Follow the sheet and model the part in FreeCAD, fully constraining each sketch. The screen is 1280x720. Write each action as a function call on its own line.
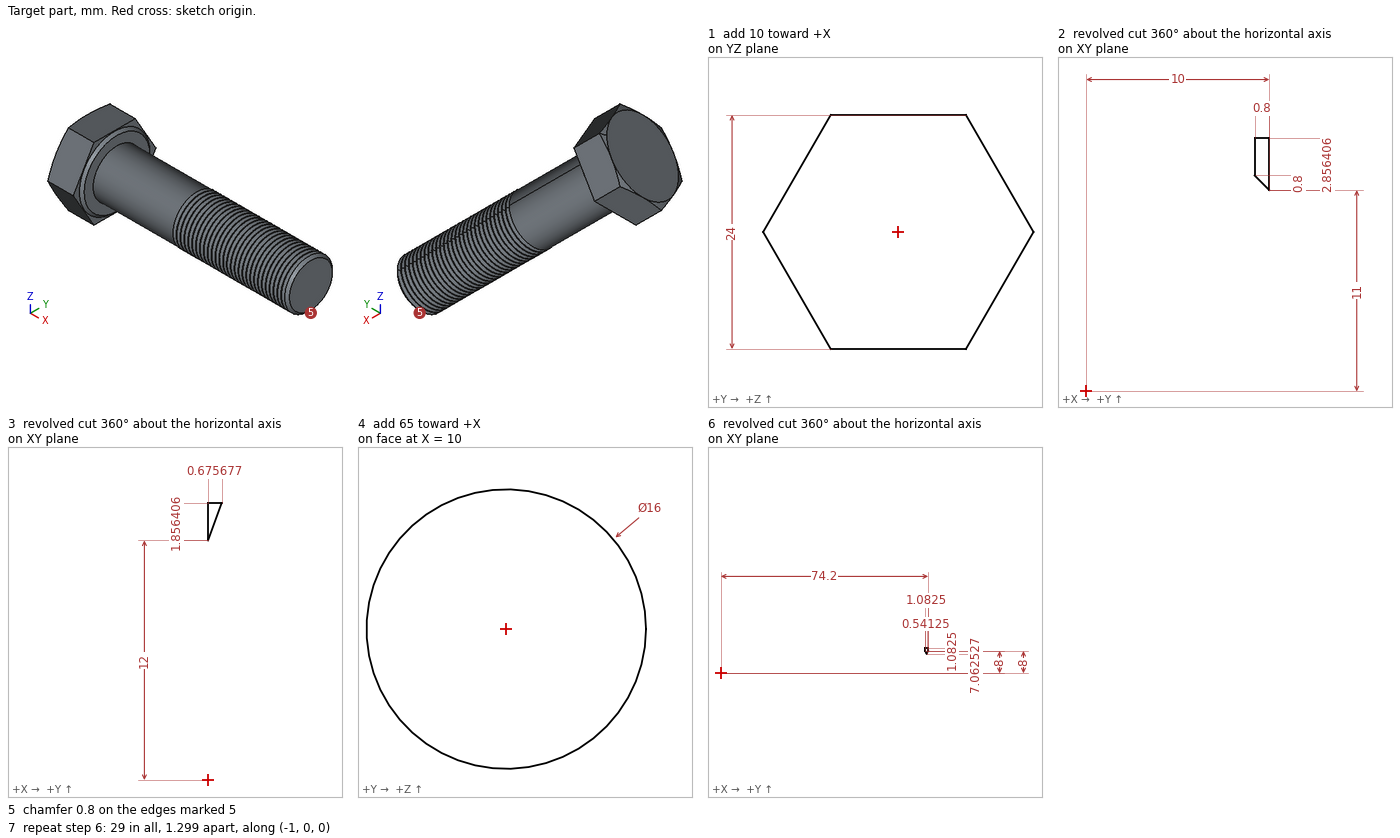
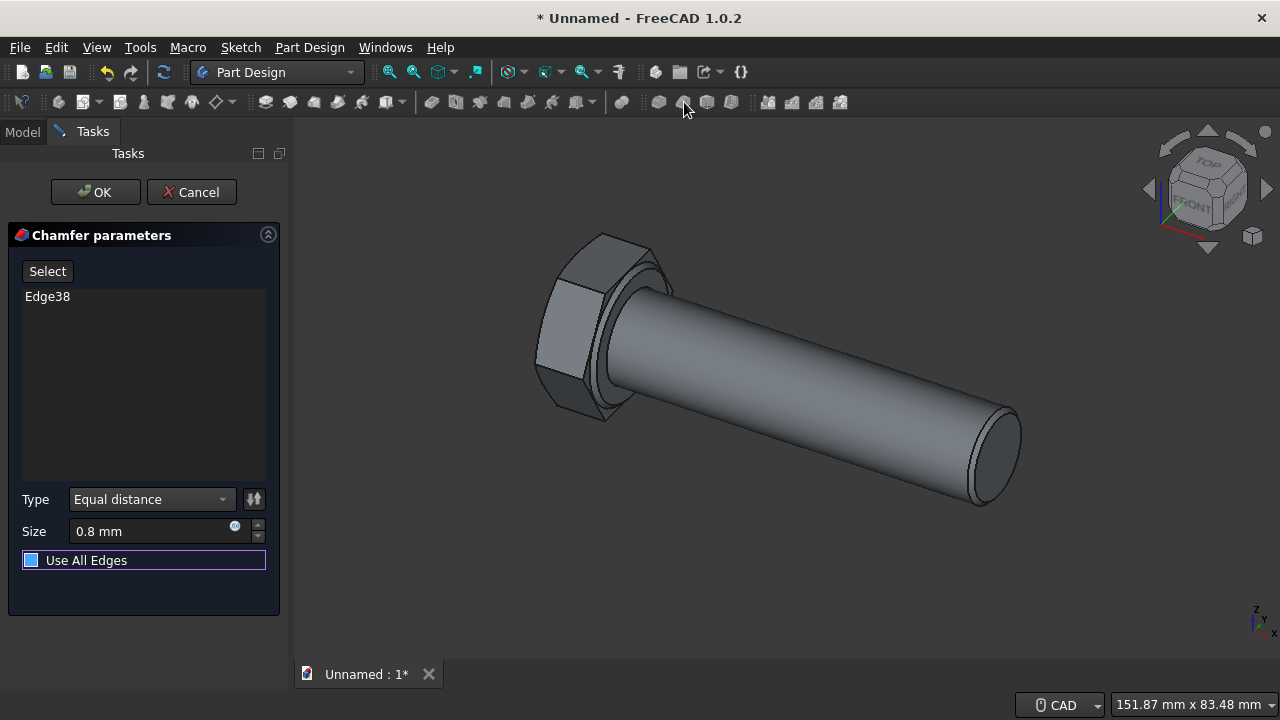
click(96, 192)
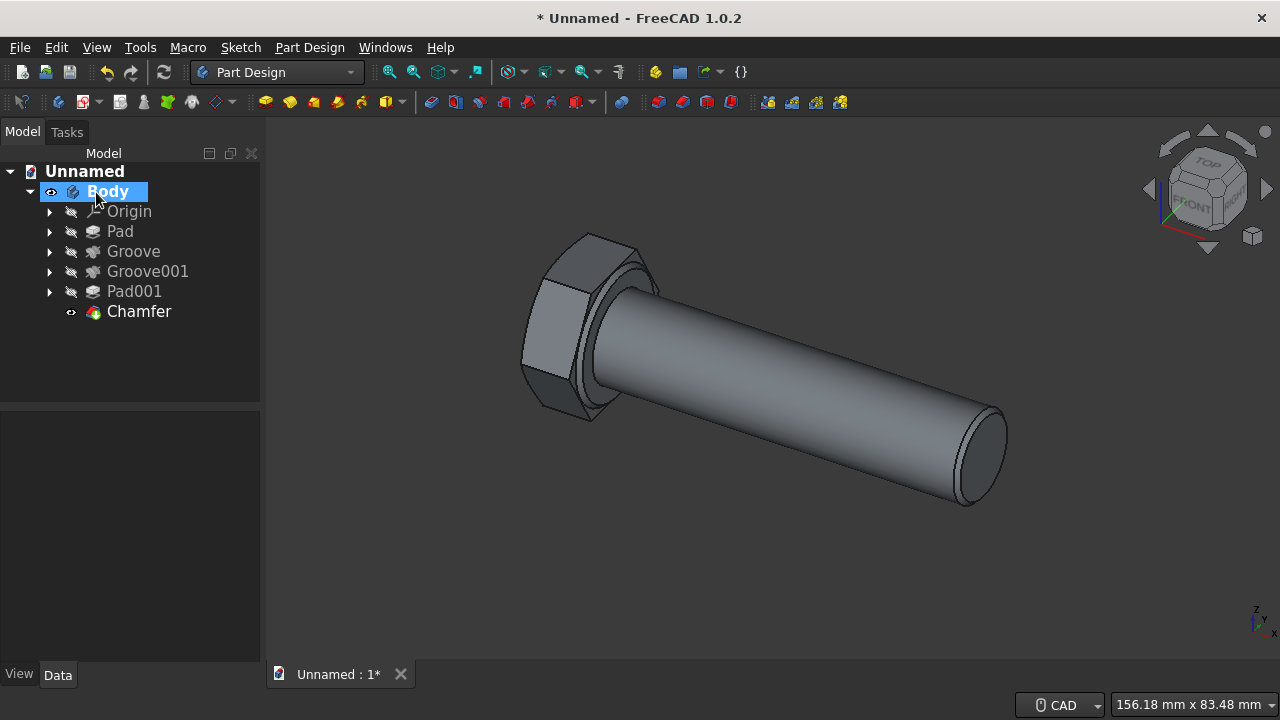
click(84, 102)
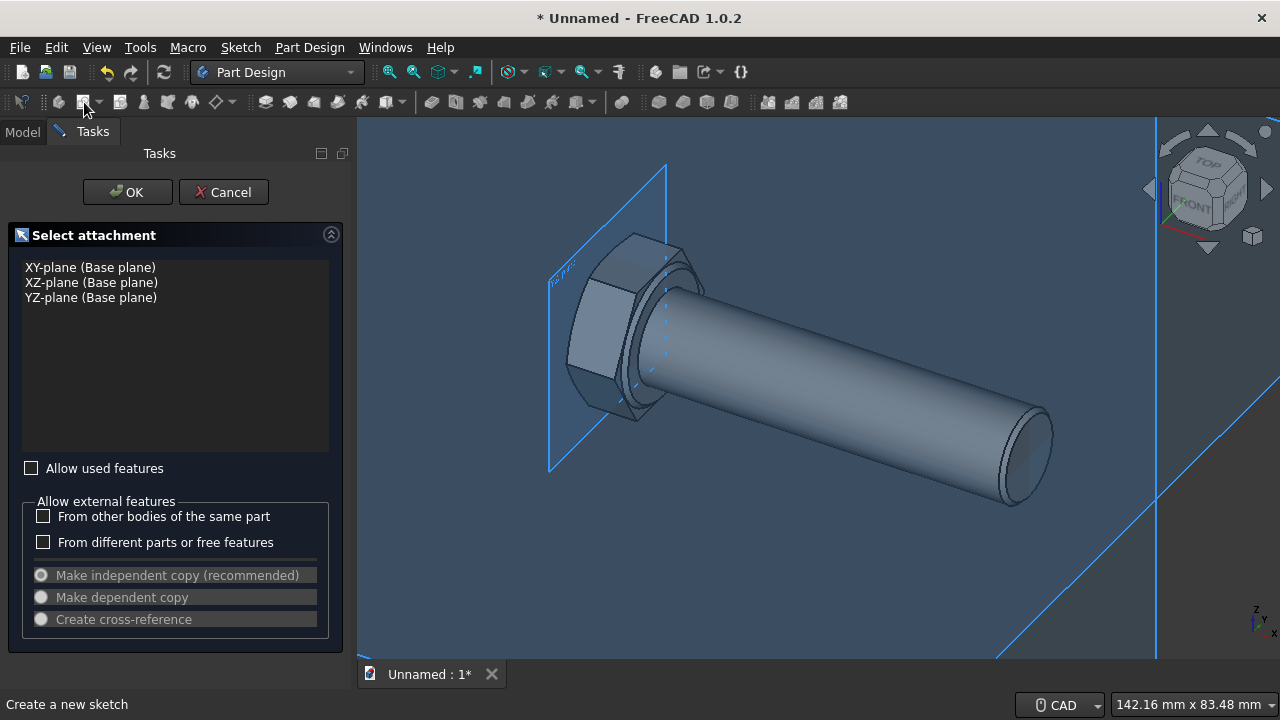
click(82, 268)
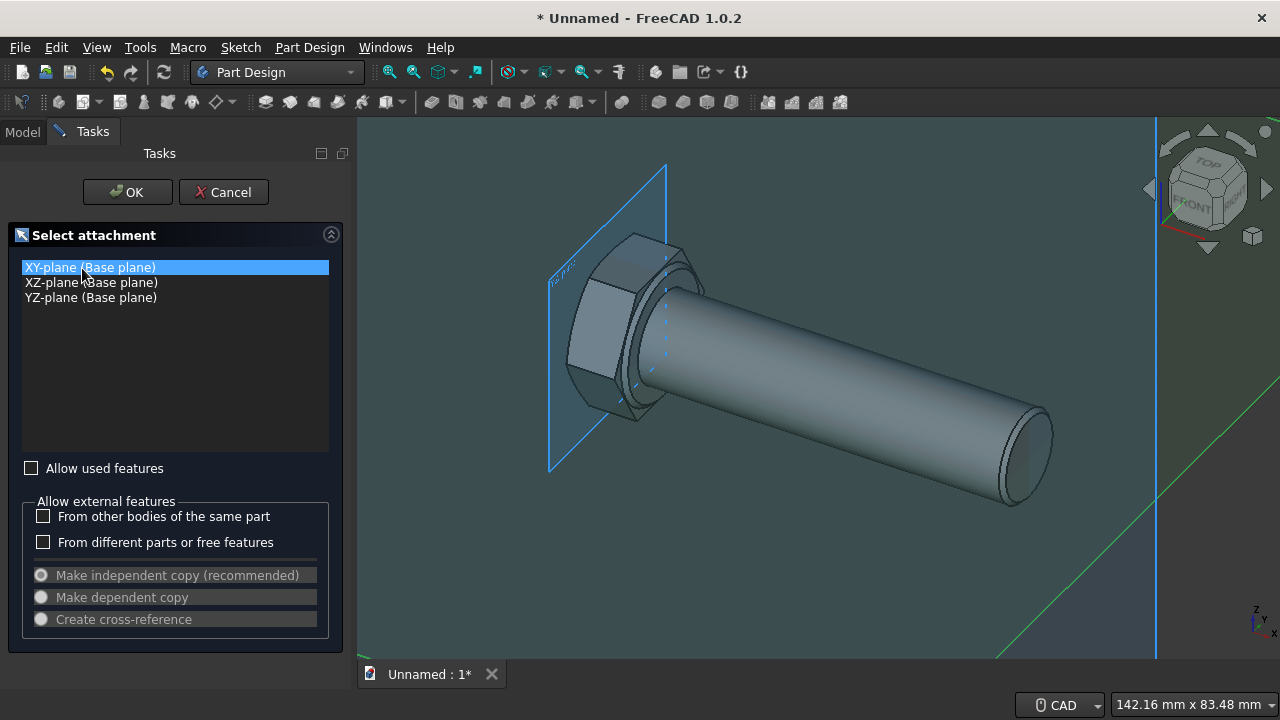
click(128, 192)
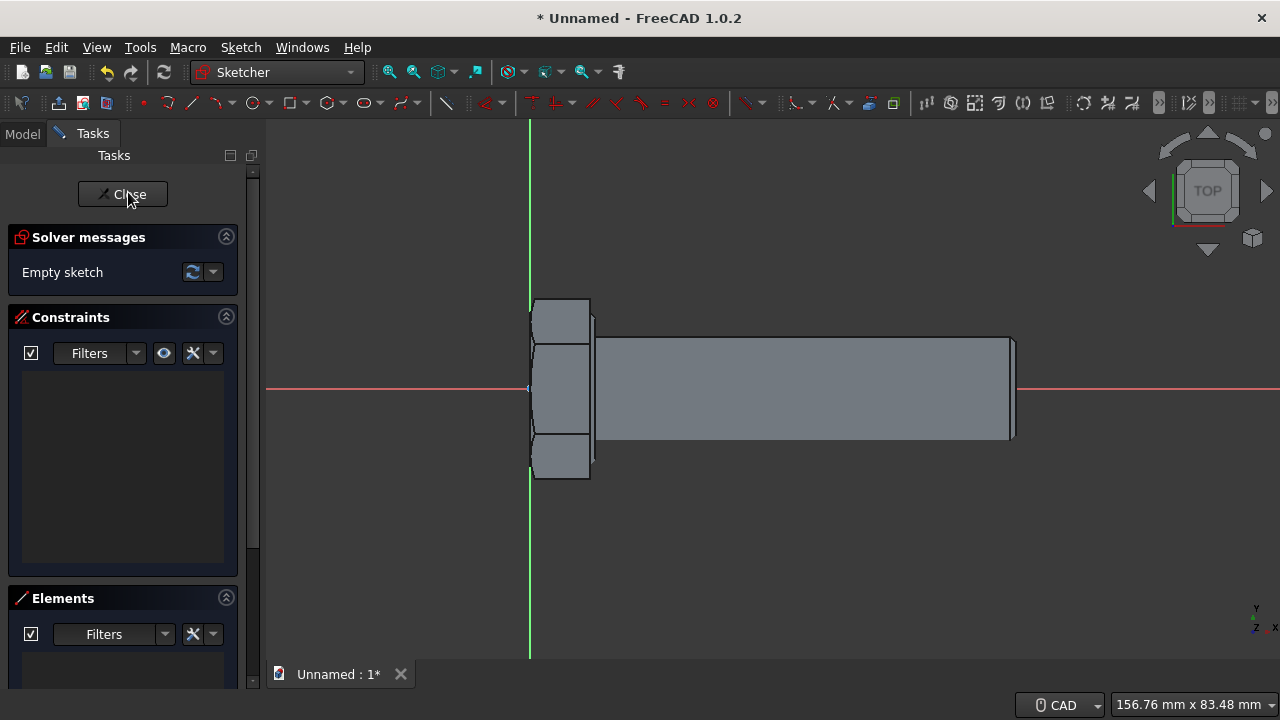
click(108, 104)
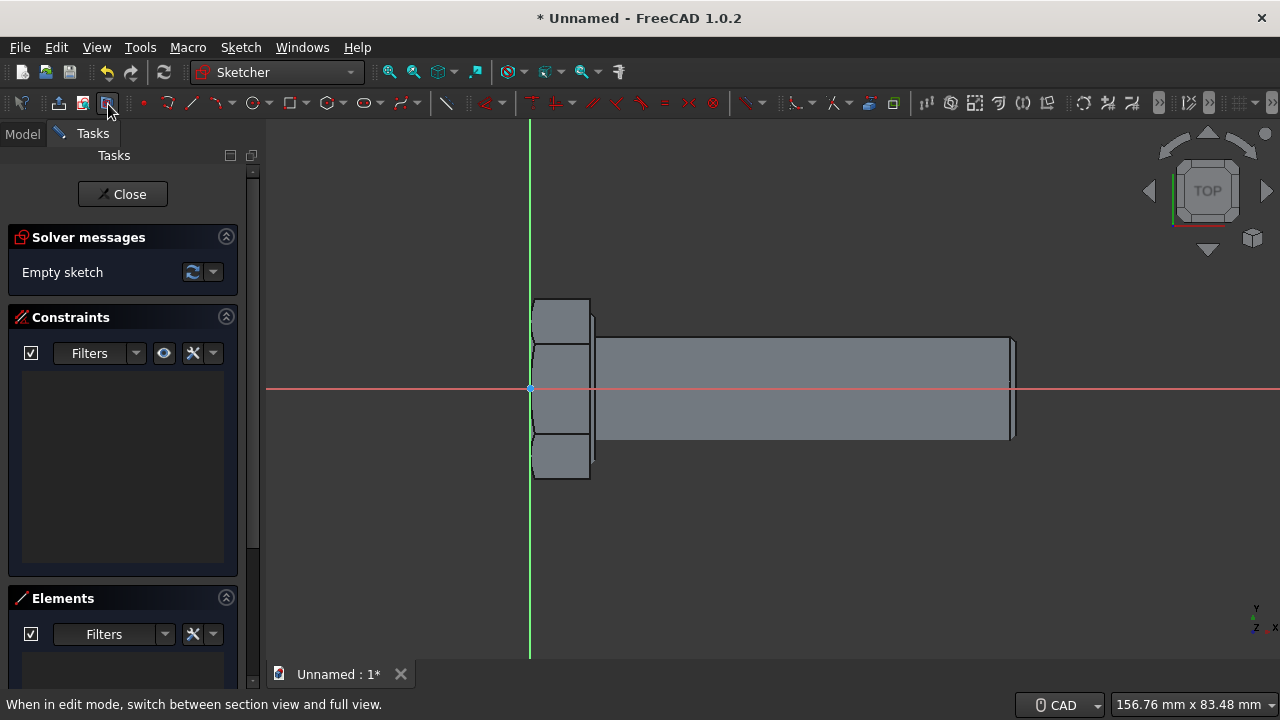
scroll(1023, 334, up, 15)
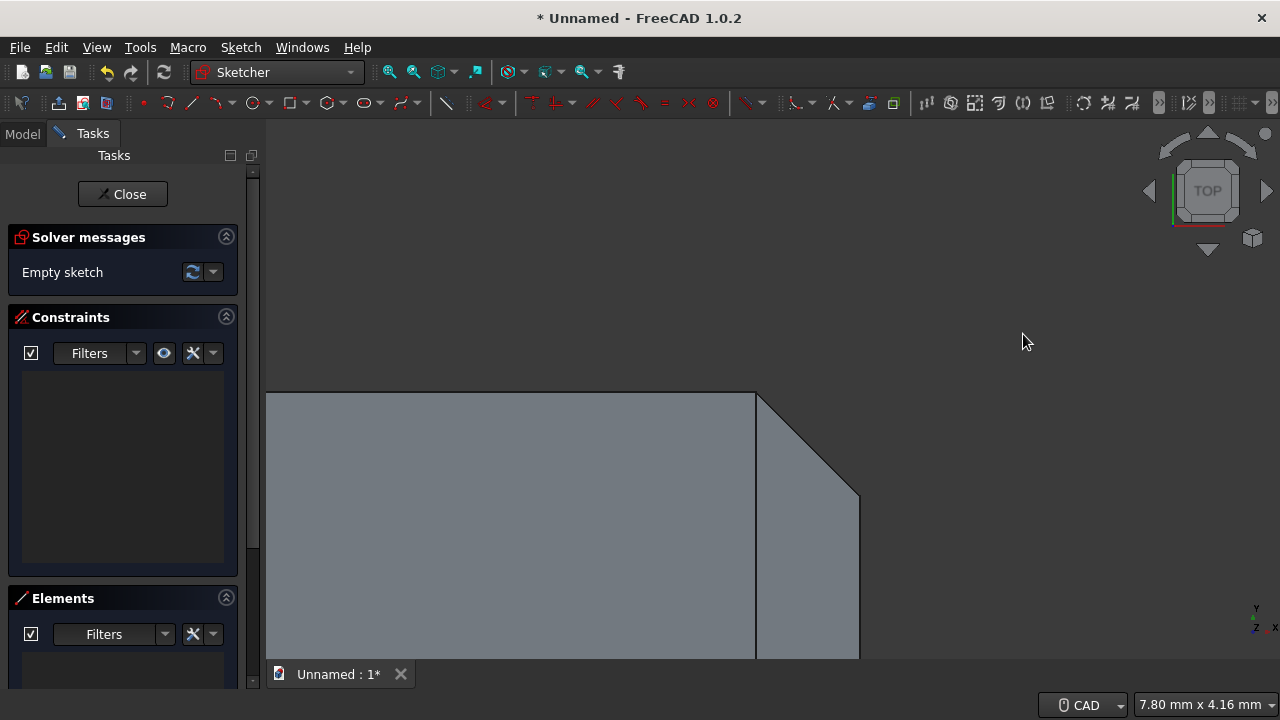
click(168, 104)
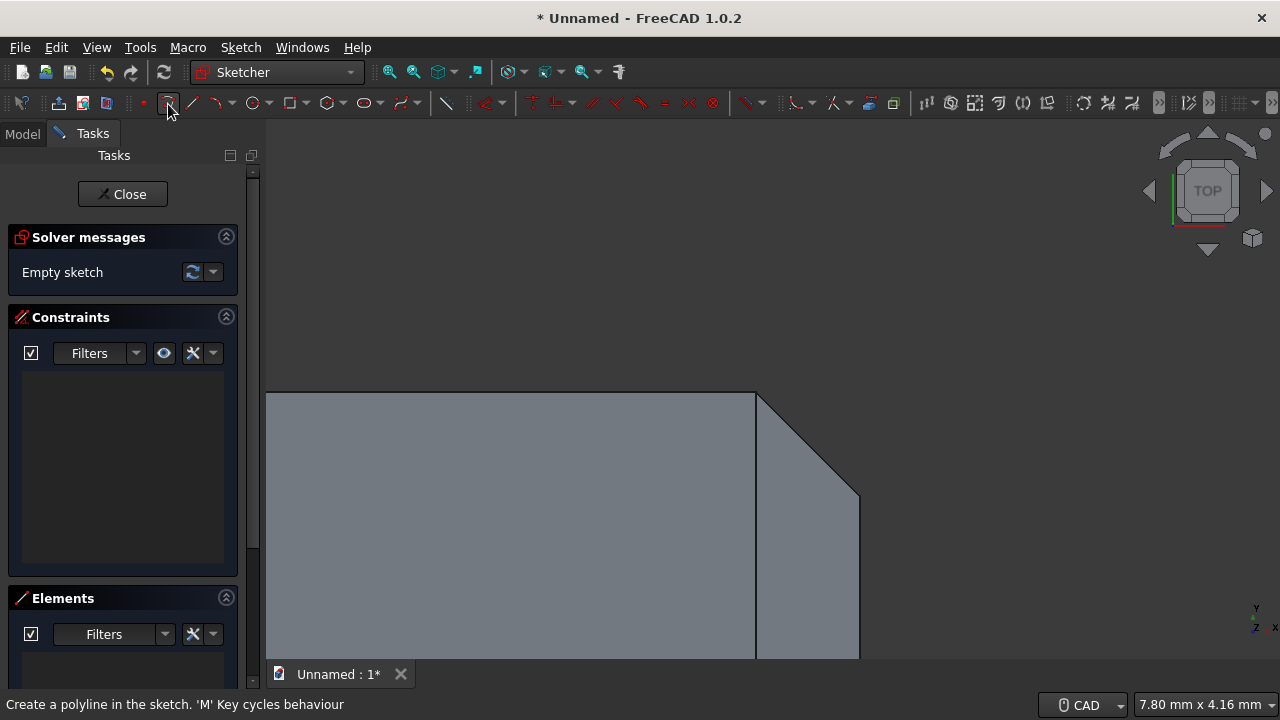
click(615, 392)
click(685, 513)
click(756, 392)
click(756, 251)
click(615, 251)
click(615, 393)
key(Escape)
key(Escape)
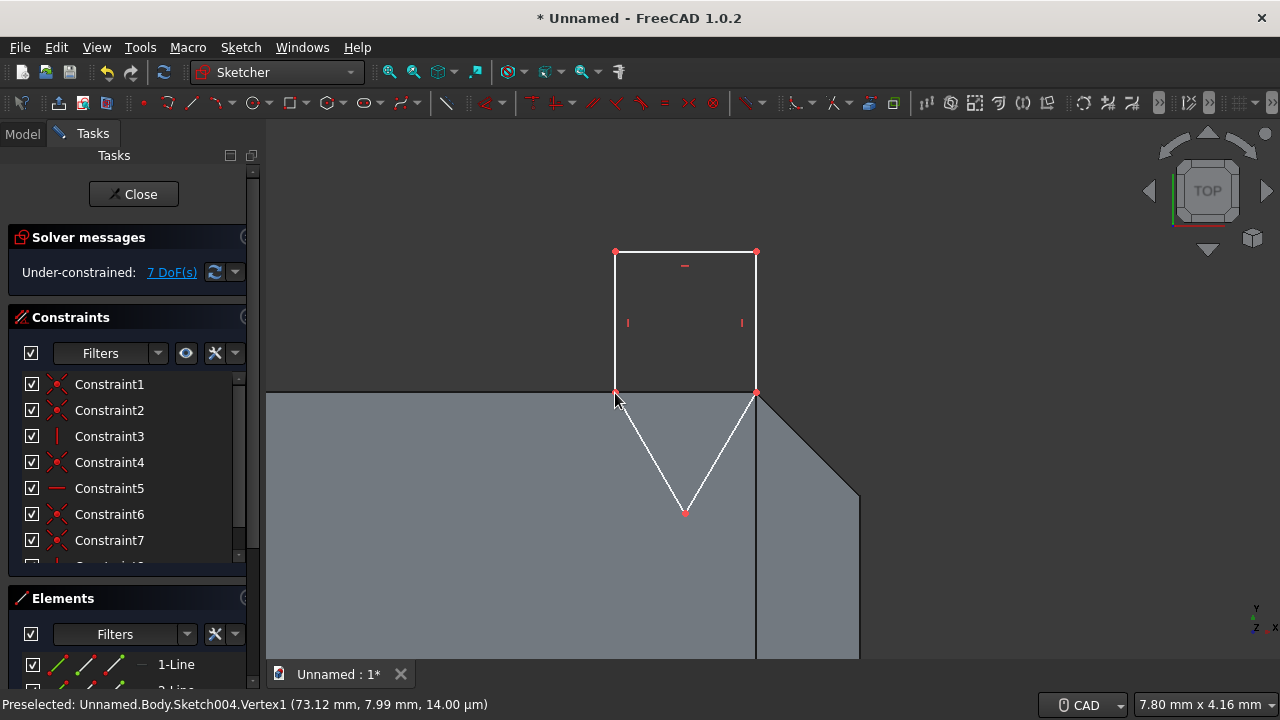
click(486, 104)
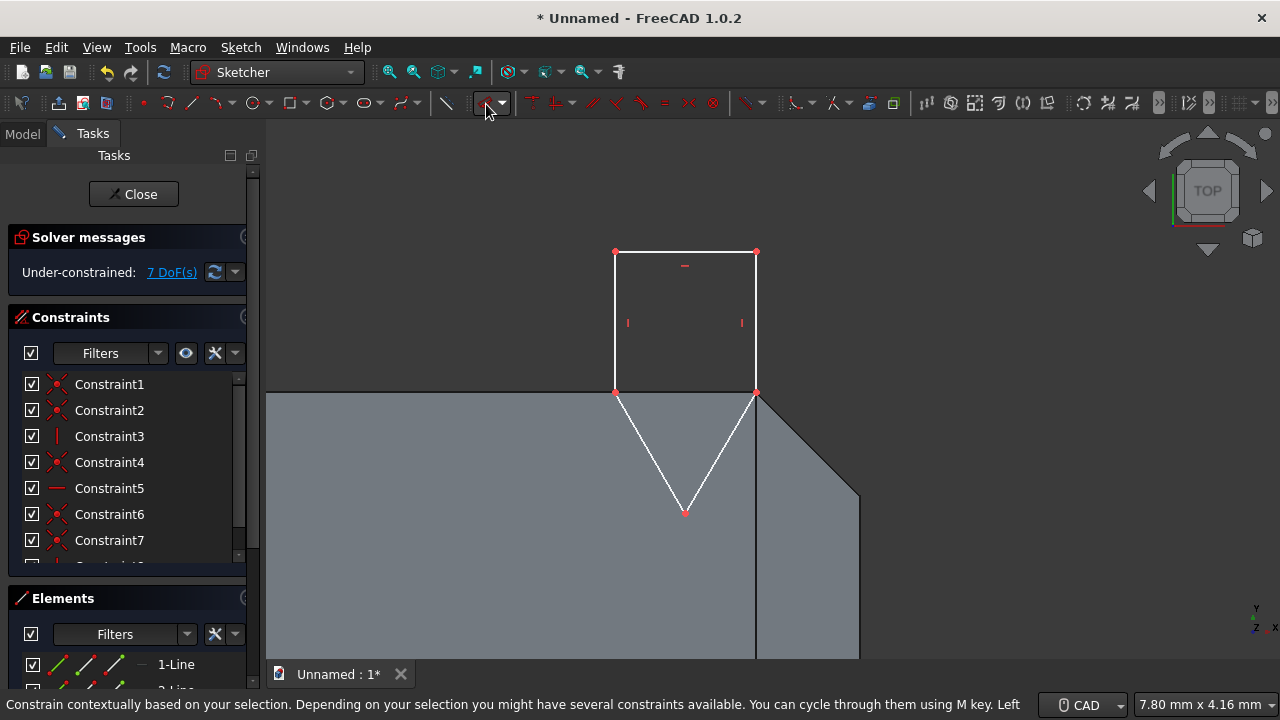
click(615, 393)
click(649, 512)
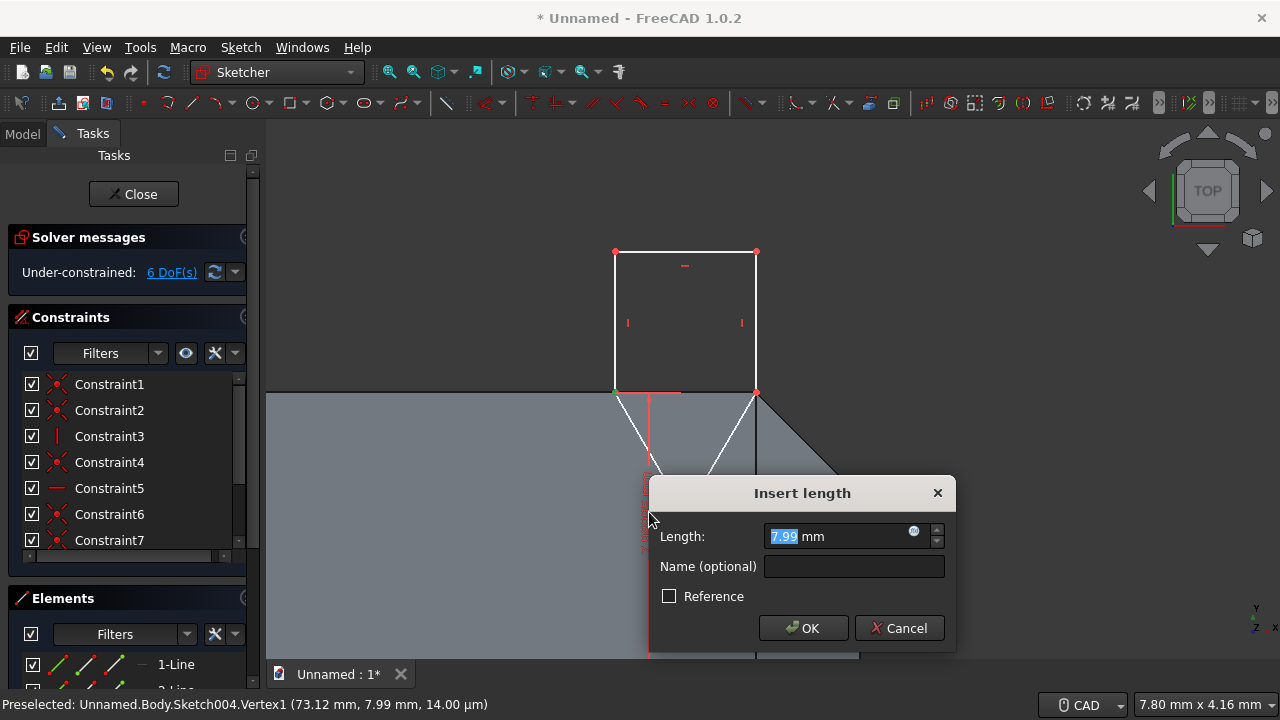
text(8)
key(Return)